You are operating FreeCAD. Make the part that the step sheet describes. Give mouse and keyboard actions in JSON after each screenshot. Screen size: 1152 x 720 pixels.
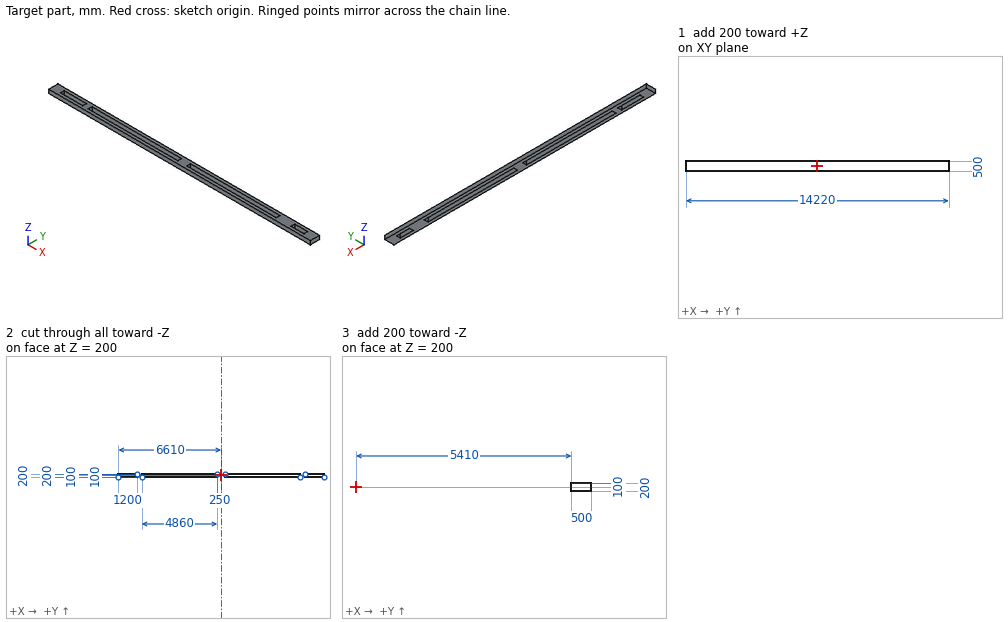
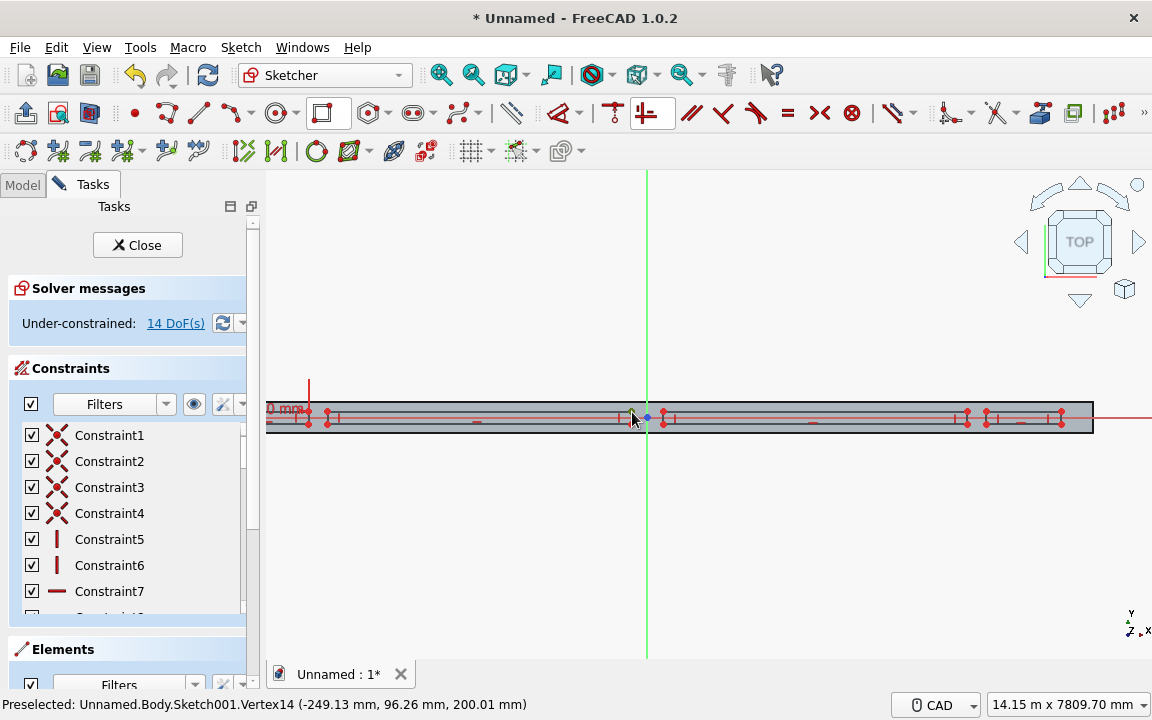
{"action": "left_click", "coordinate": [663, 412]}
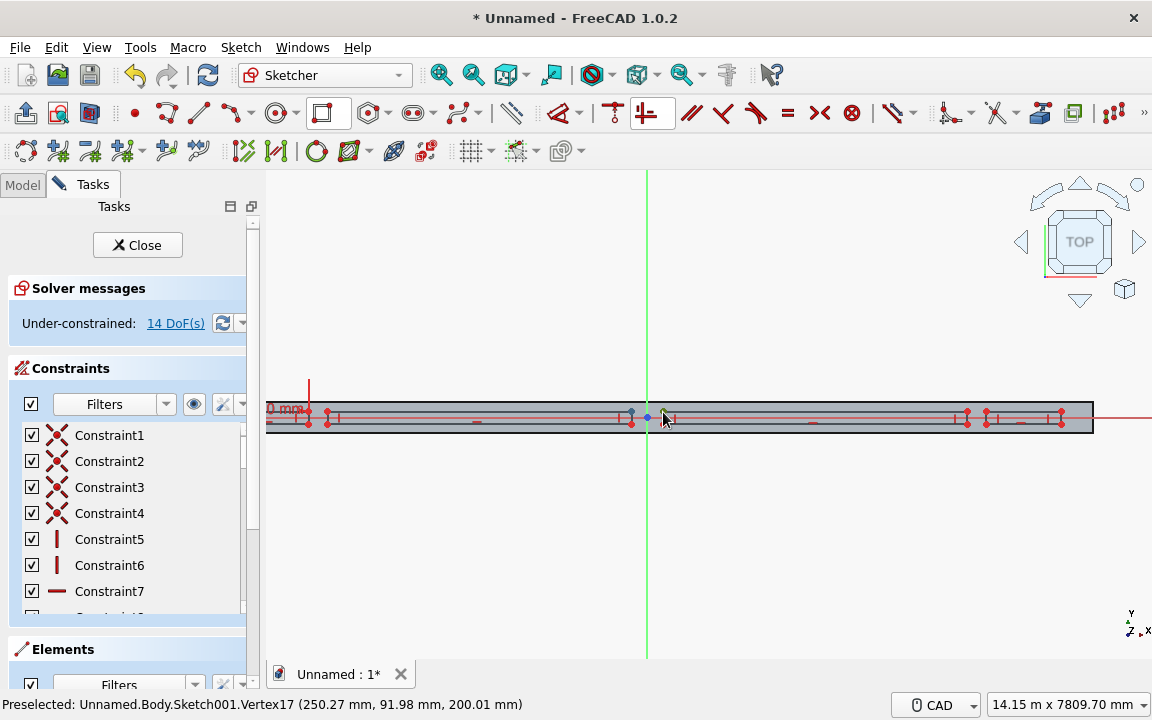
{"action": "left_click", "coordinate": [647, 600]}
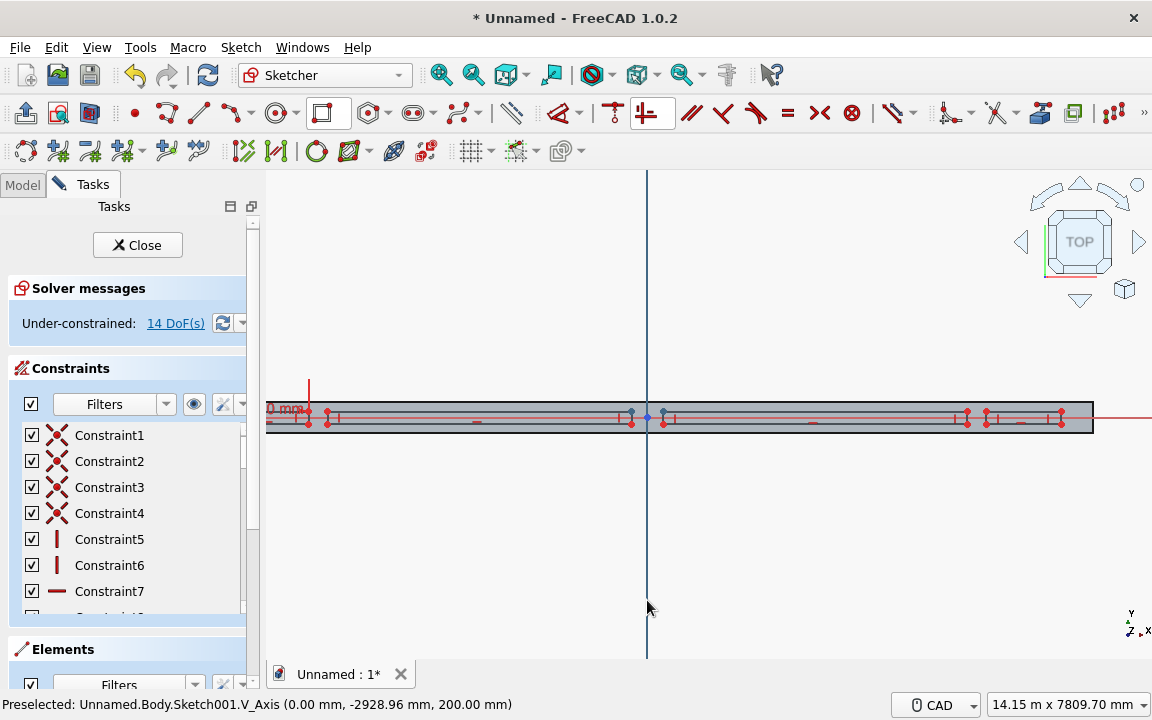
{"action": "left_click", "coordinate": [820, 114]}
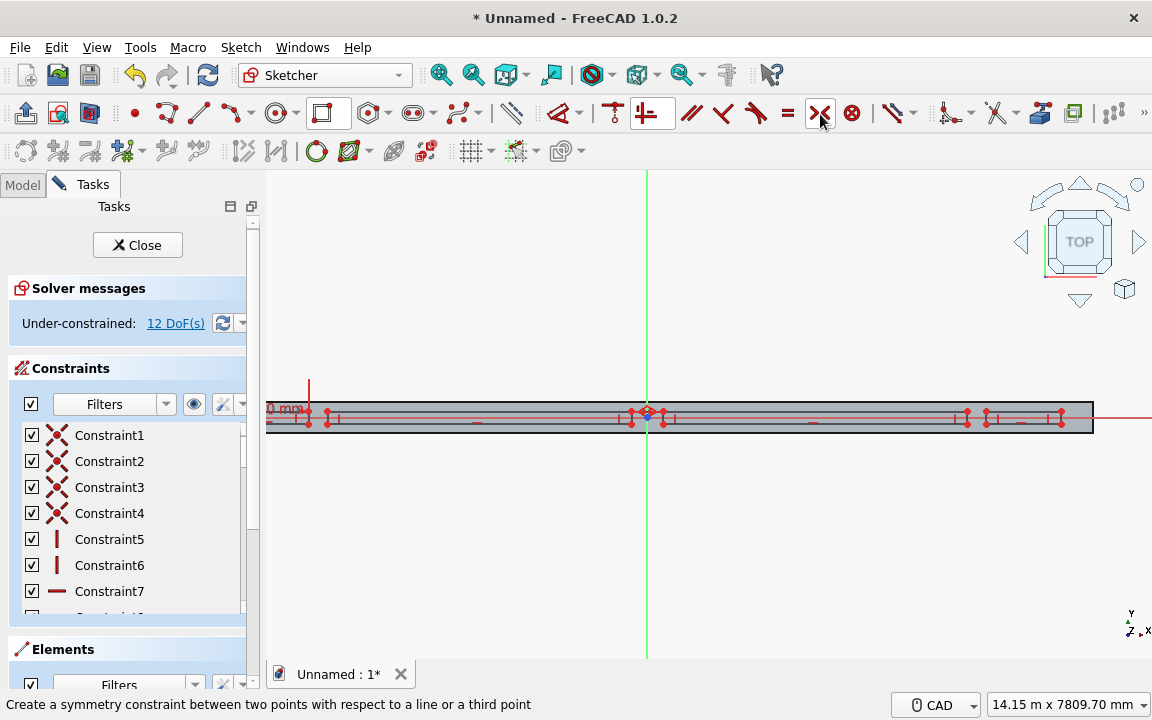
{"action": "left_click", "coordinate": [328, 424]}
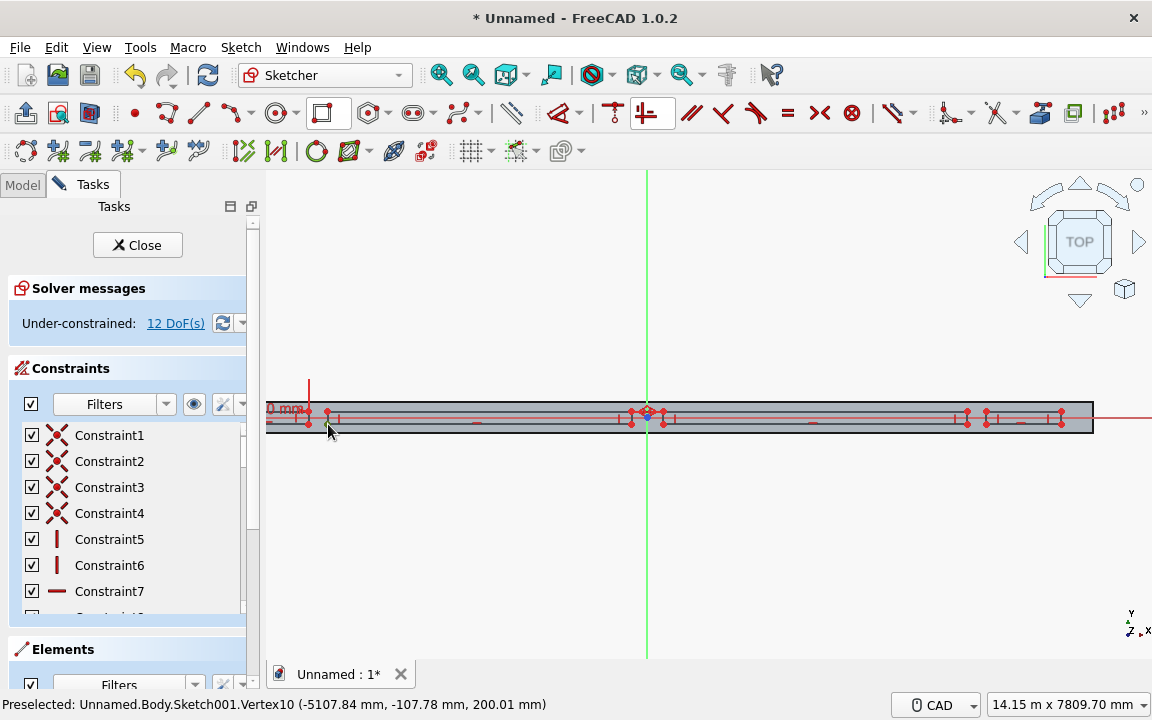
{"action": "left_click", "coordinate": [967, 424]}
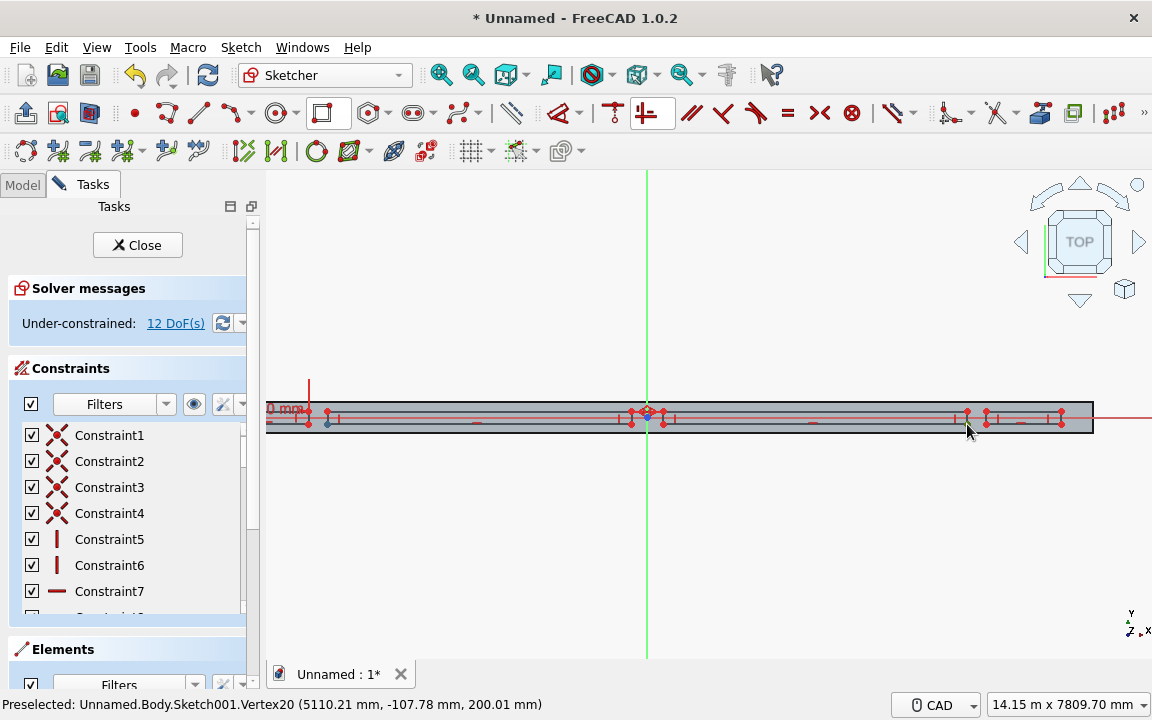
{"action": "left_click", "coordinate": [647, 600]}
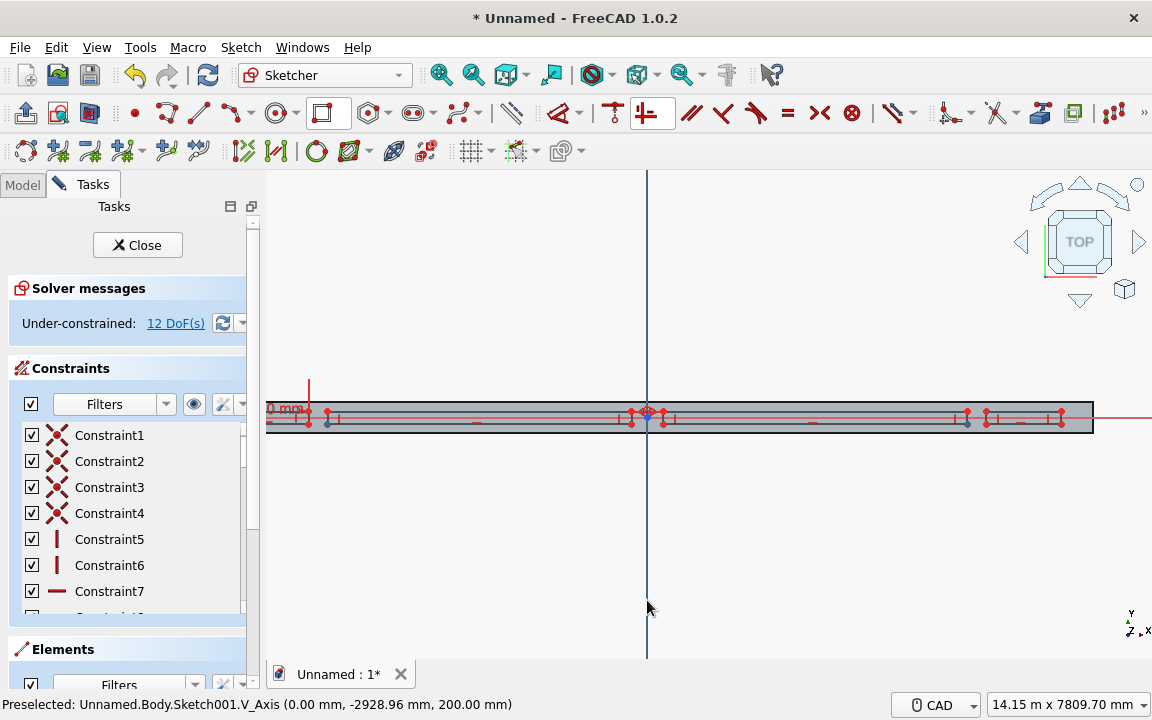
{"action": "left_click", "coordinate": [820, 114]}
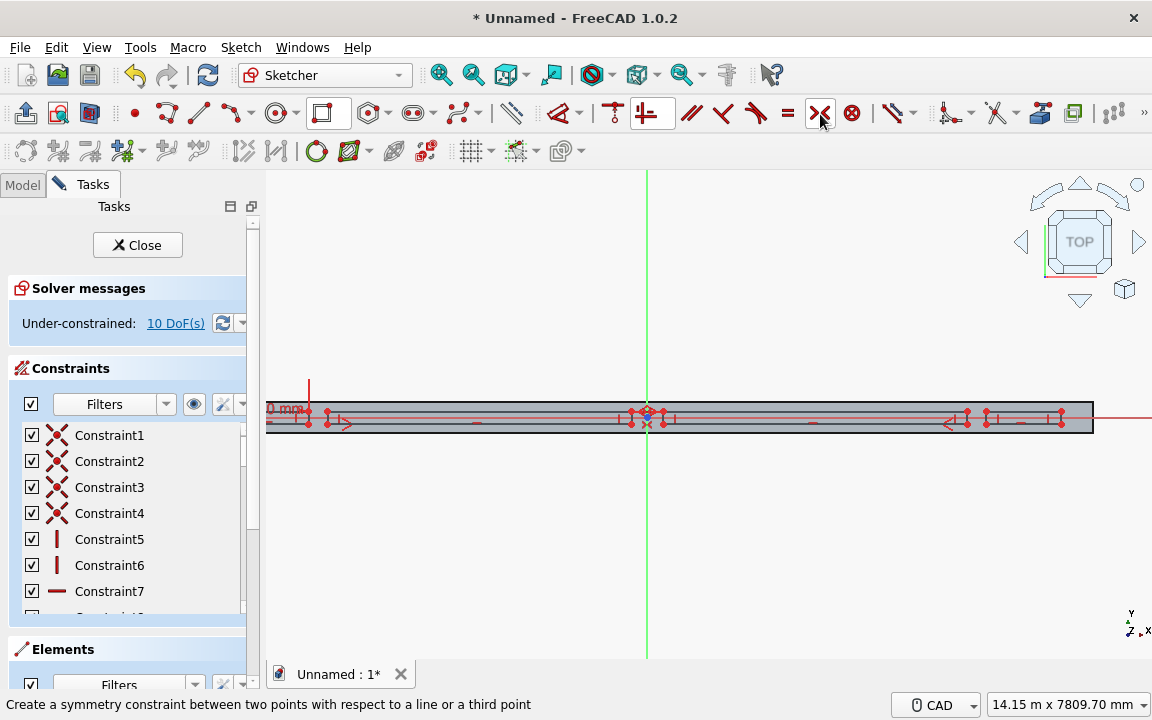
{"action": "left_click", "coordinate": [309, 412]}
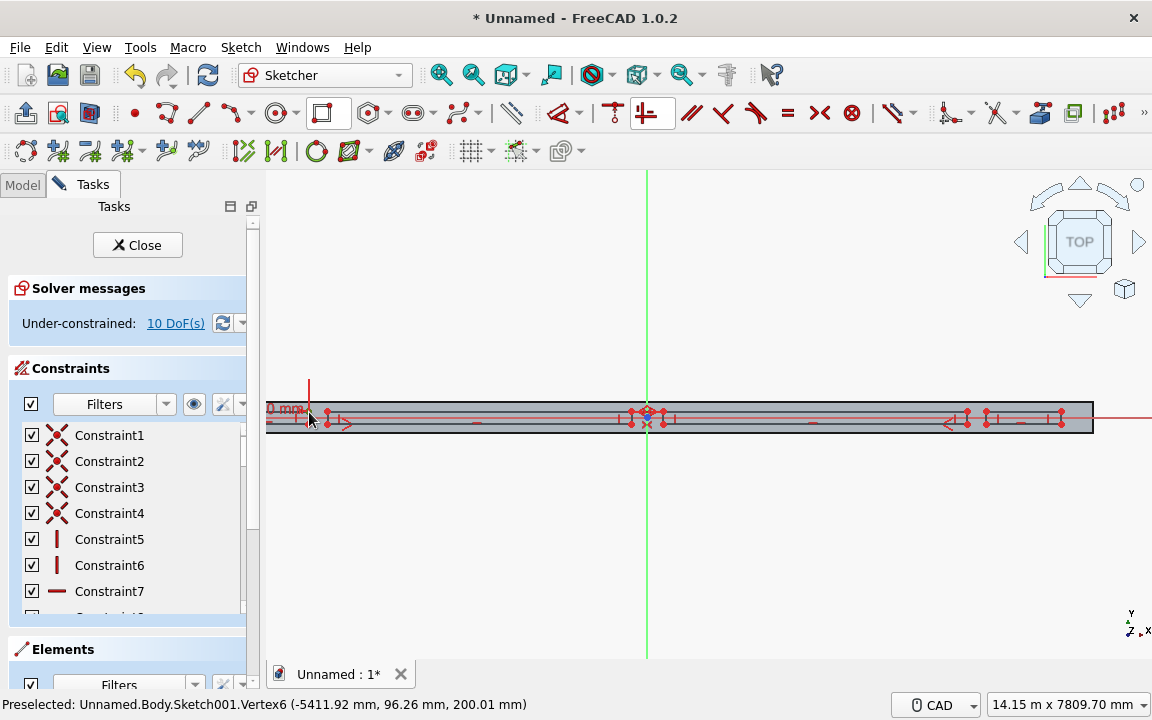
{"action": "left_click", "coordinate": [986, 412]}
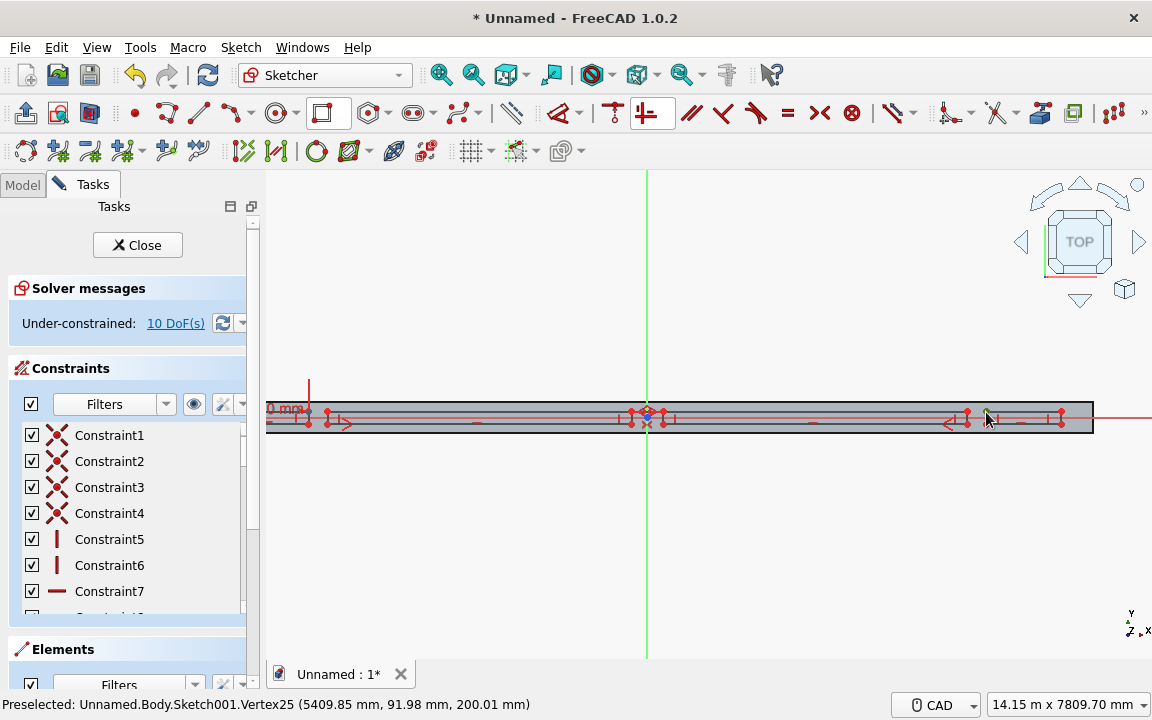
{"action": "left_click", "coordinate": [647, 600]}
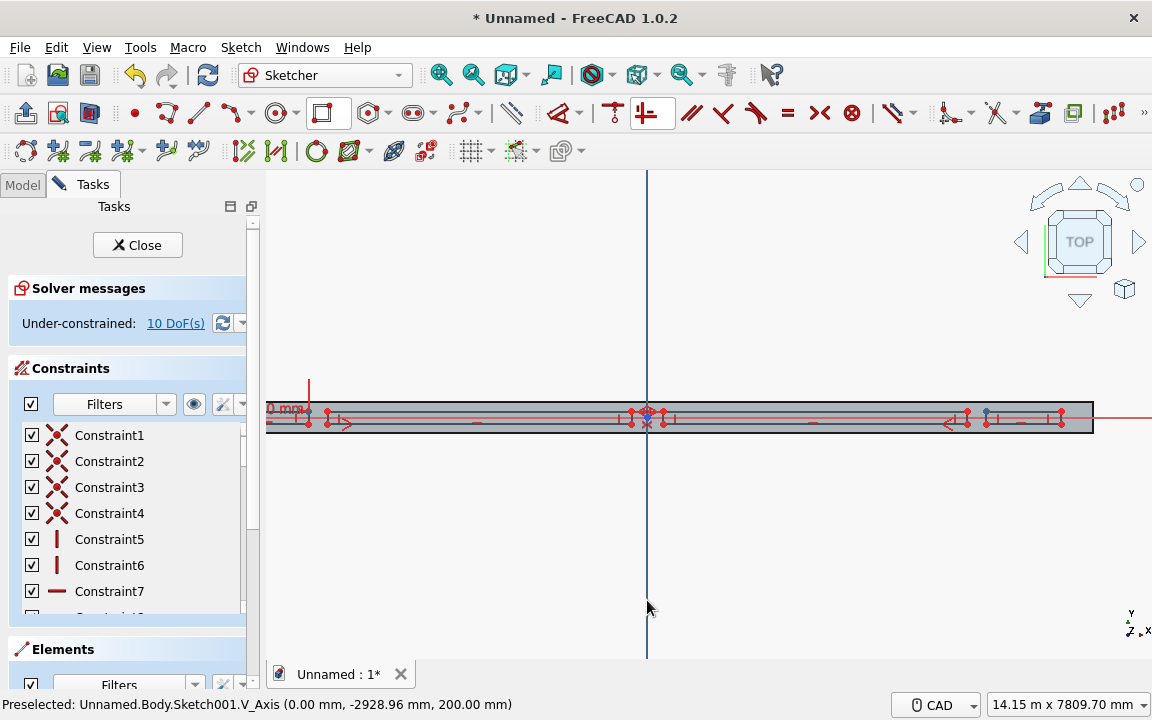
{"action": "left_click", "coordinate": [820, 114]}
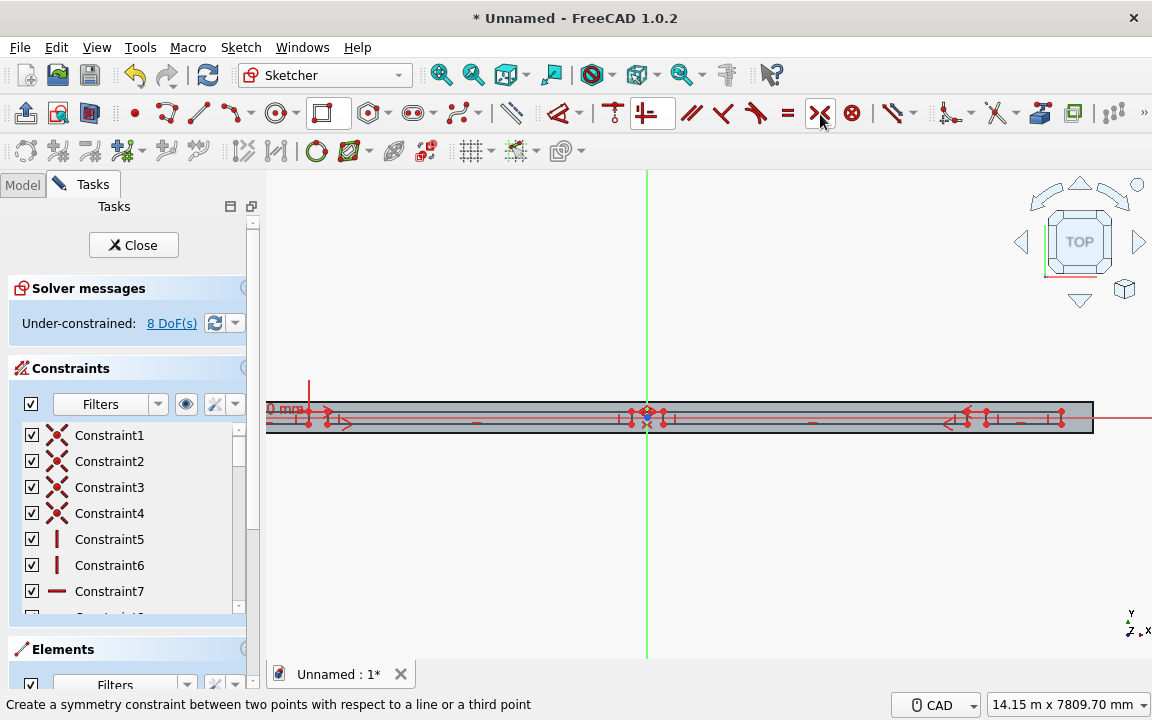
{"action": "scroll", "coordinate": [632, 411], "scroll_direction": "down", "scroll_amount": 3}